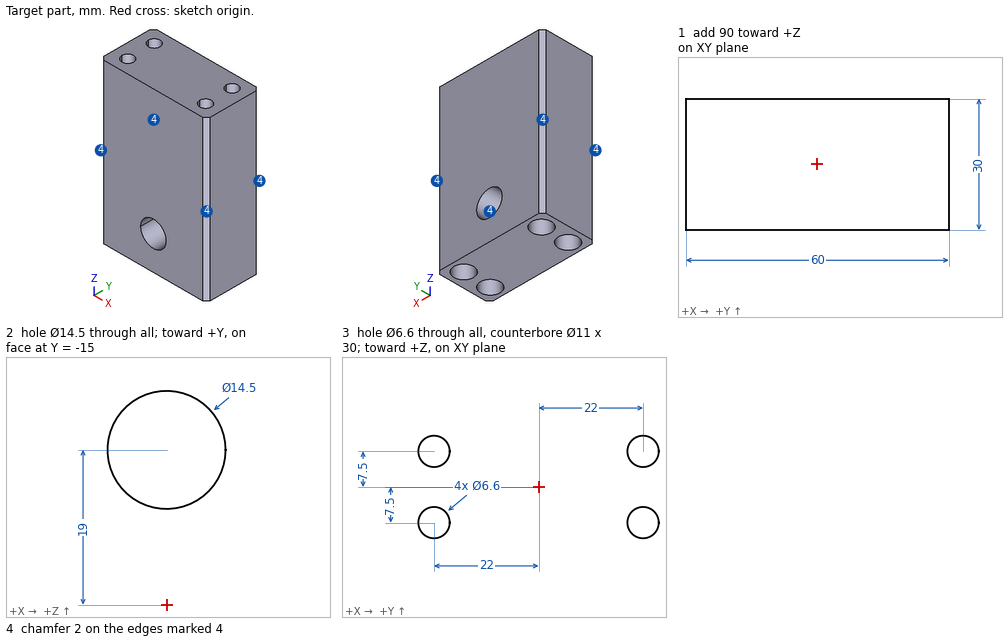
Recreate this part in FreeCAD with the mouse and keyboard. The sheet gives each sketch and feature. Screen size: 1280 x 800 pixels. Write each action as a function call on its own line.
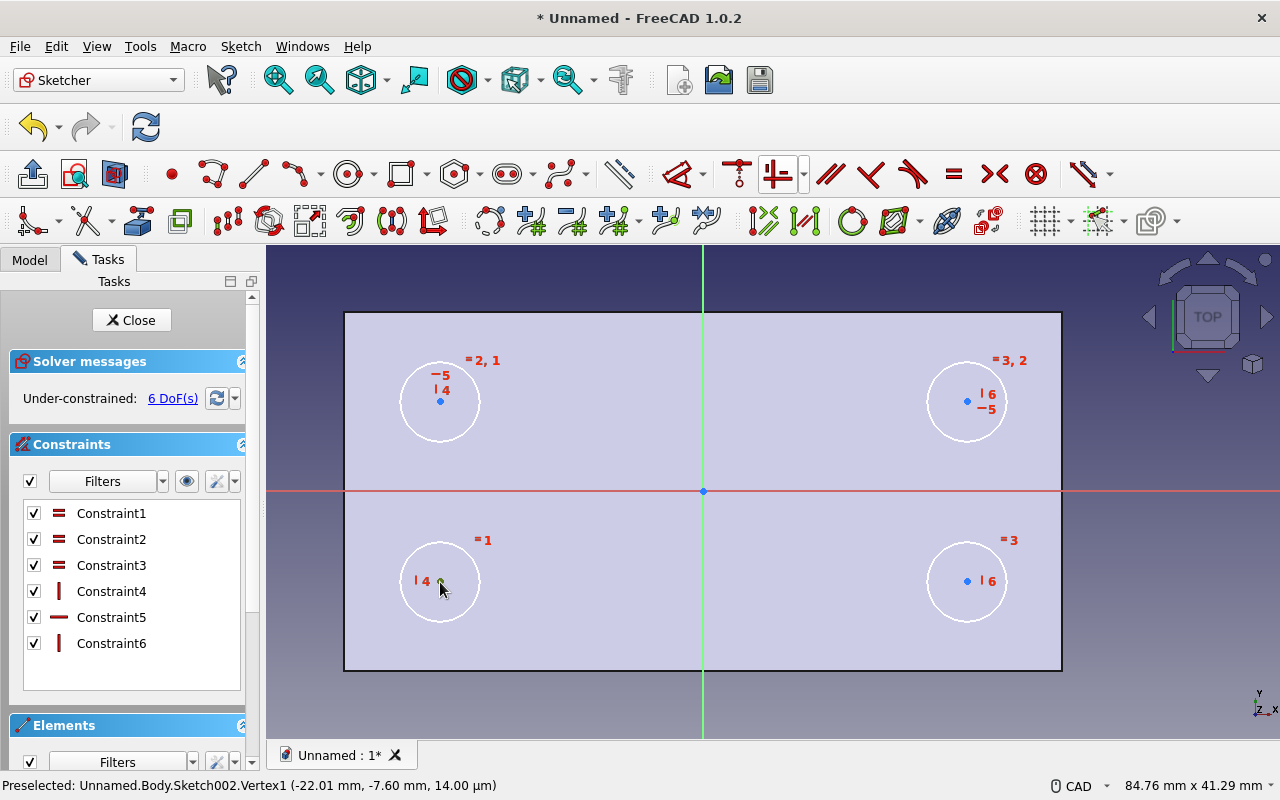
click(967, 582)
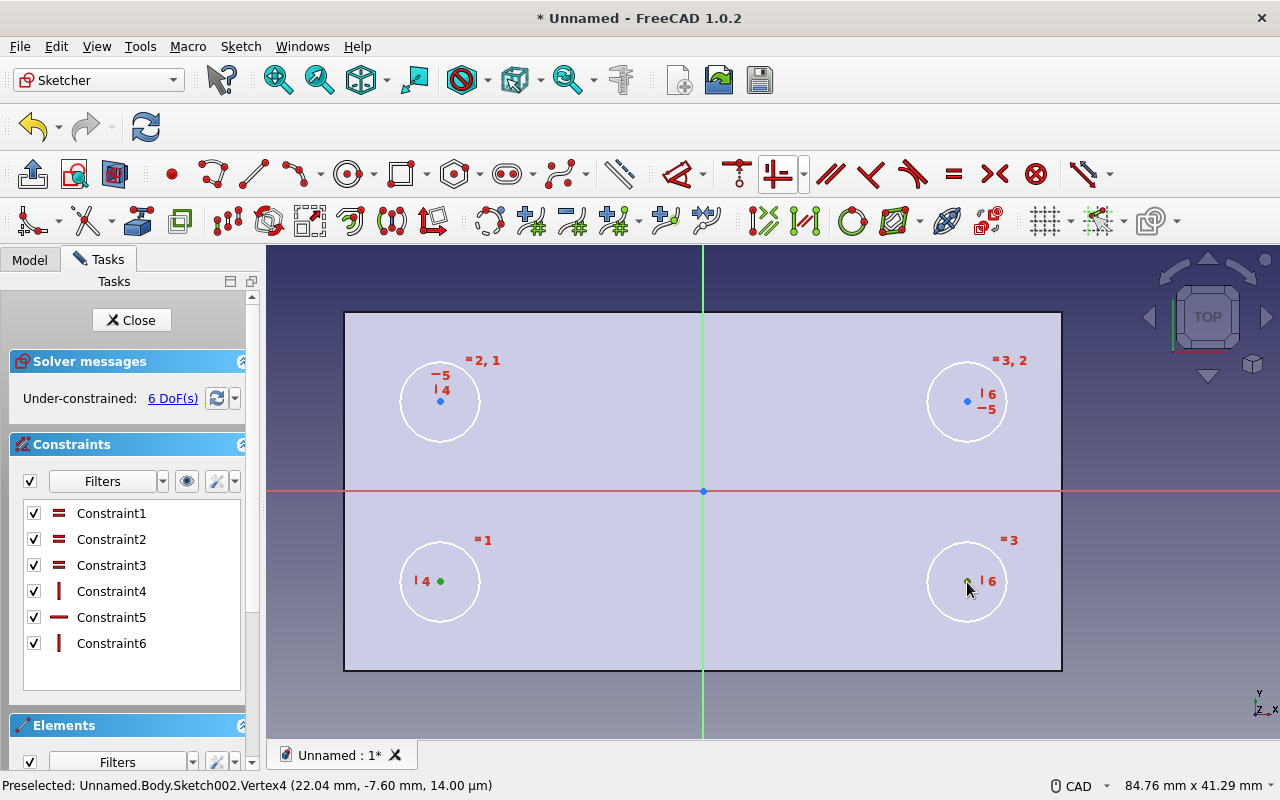
key(h)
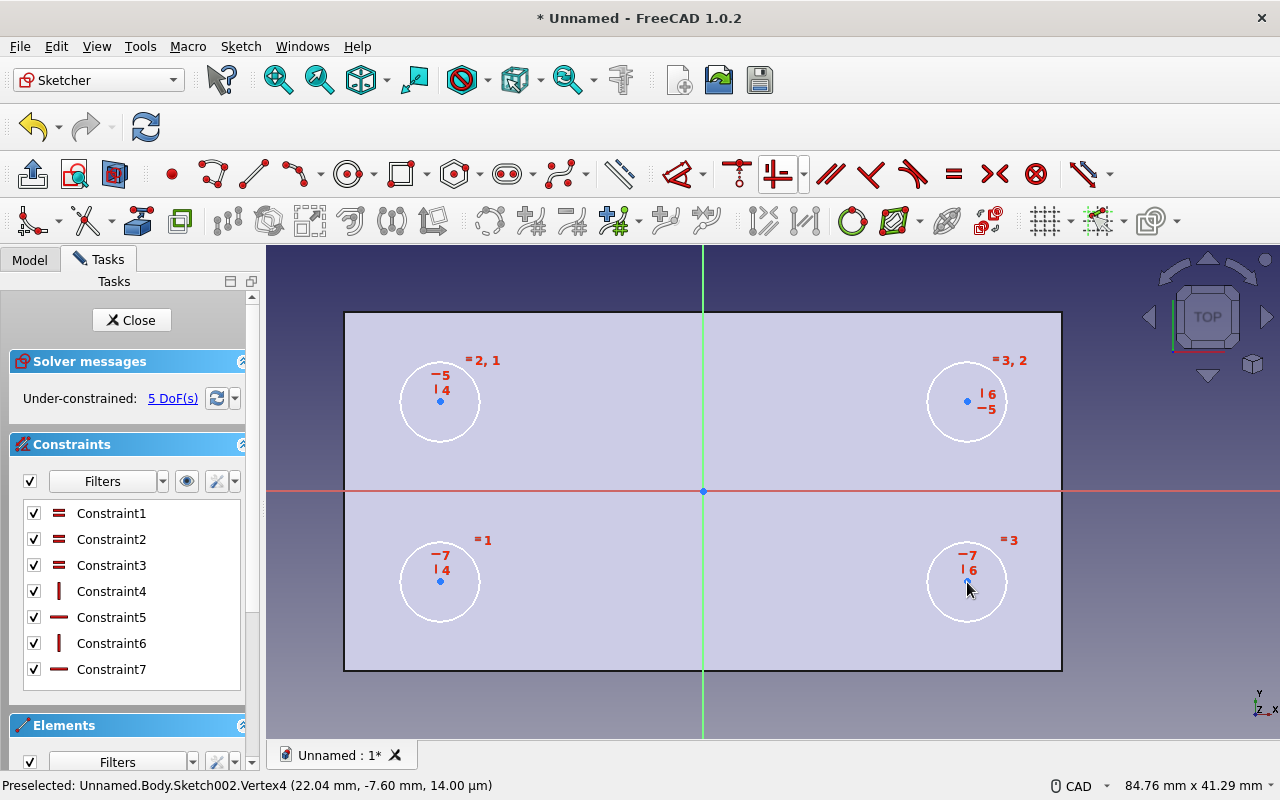
key(d)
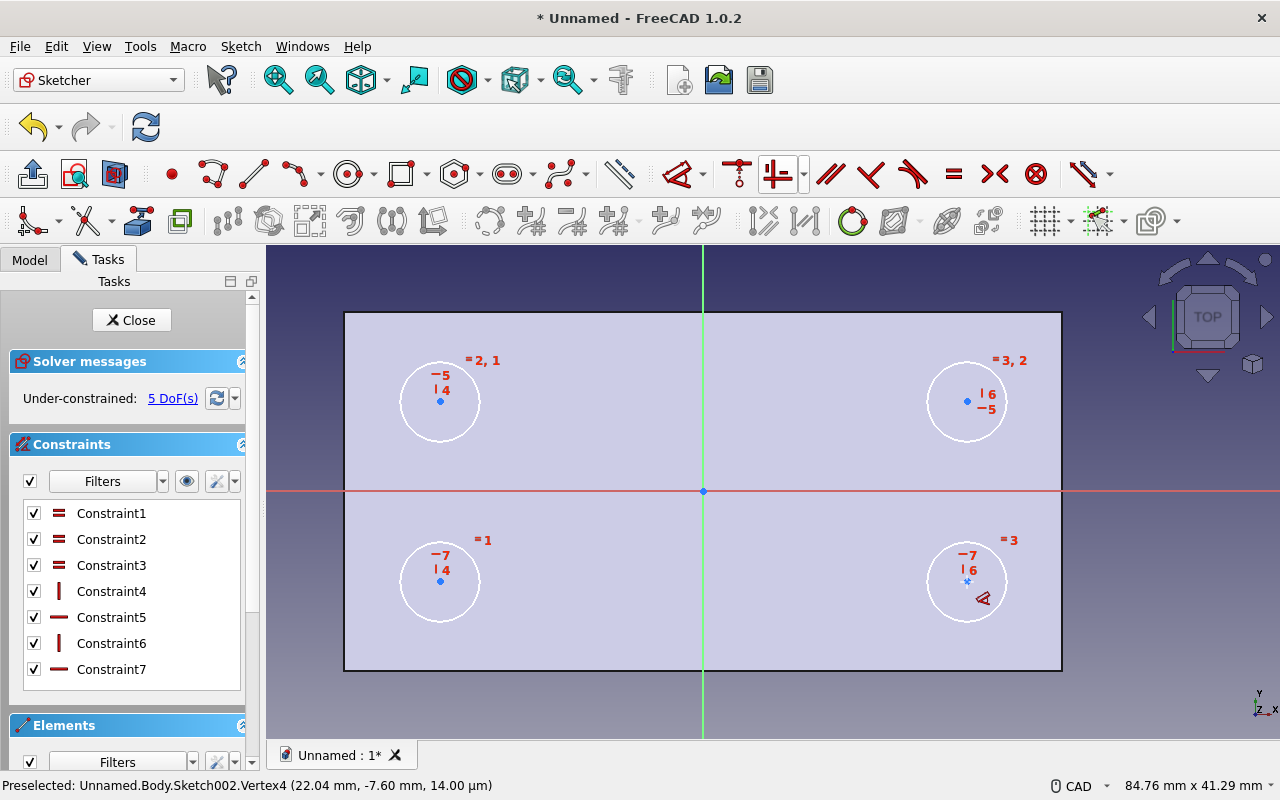
click(468, 554)
click(491, 531)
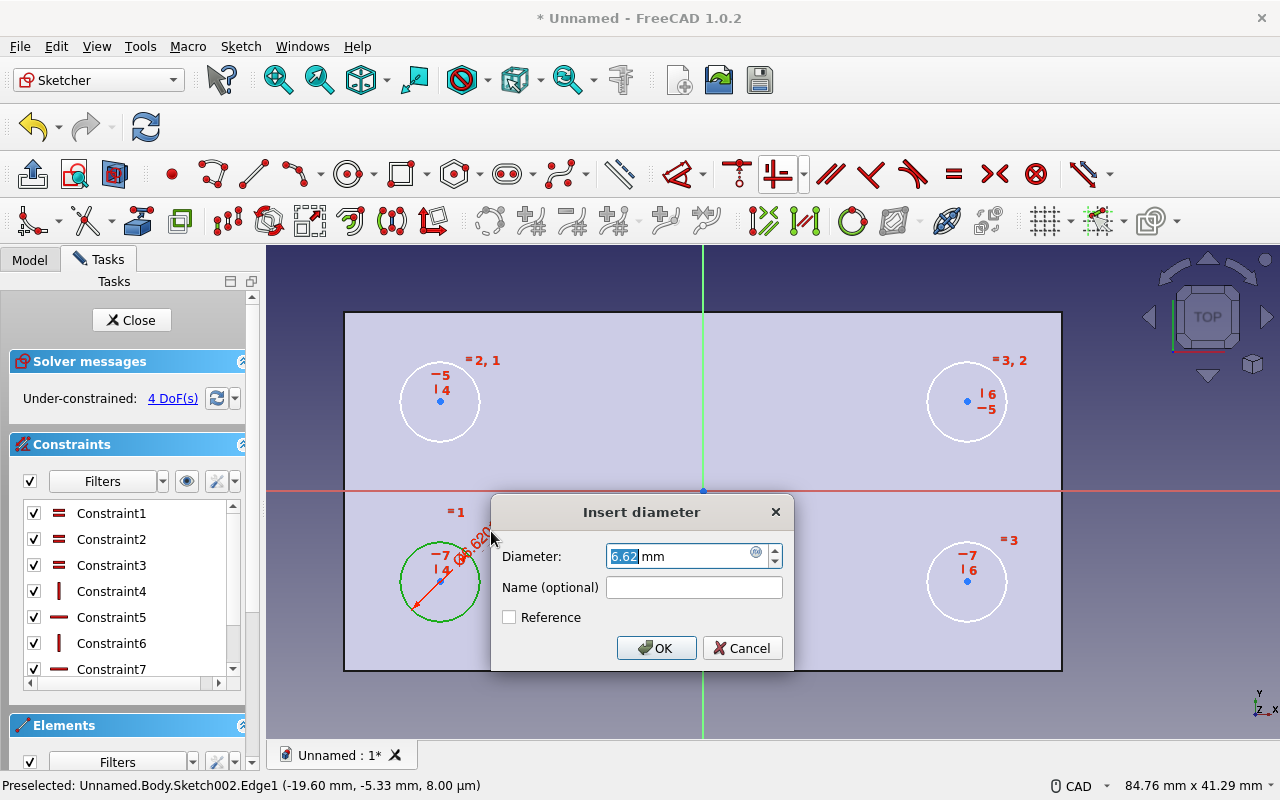
text(6.6)
key(Return)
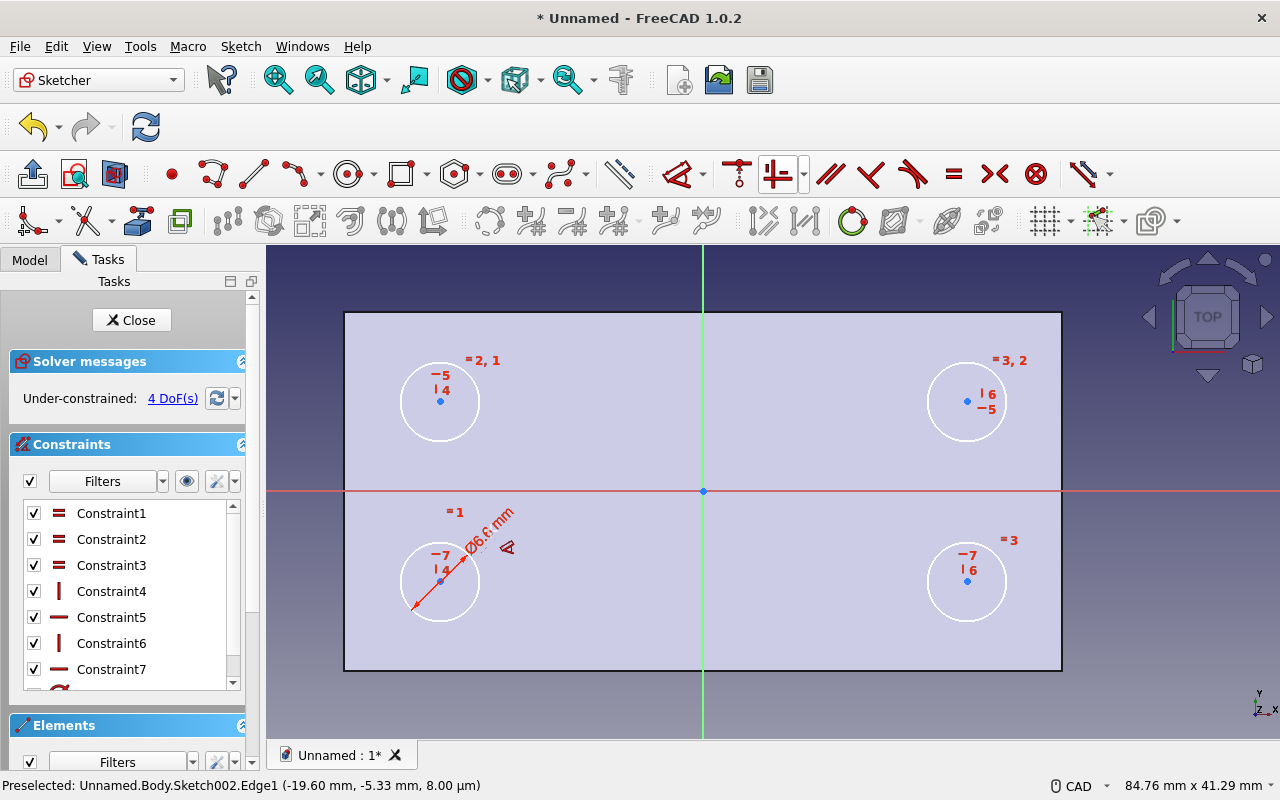
click(440, 582)
click(572, 616)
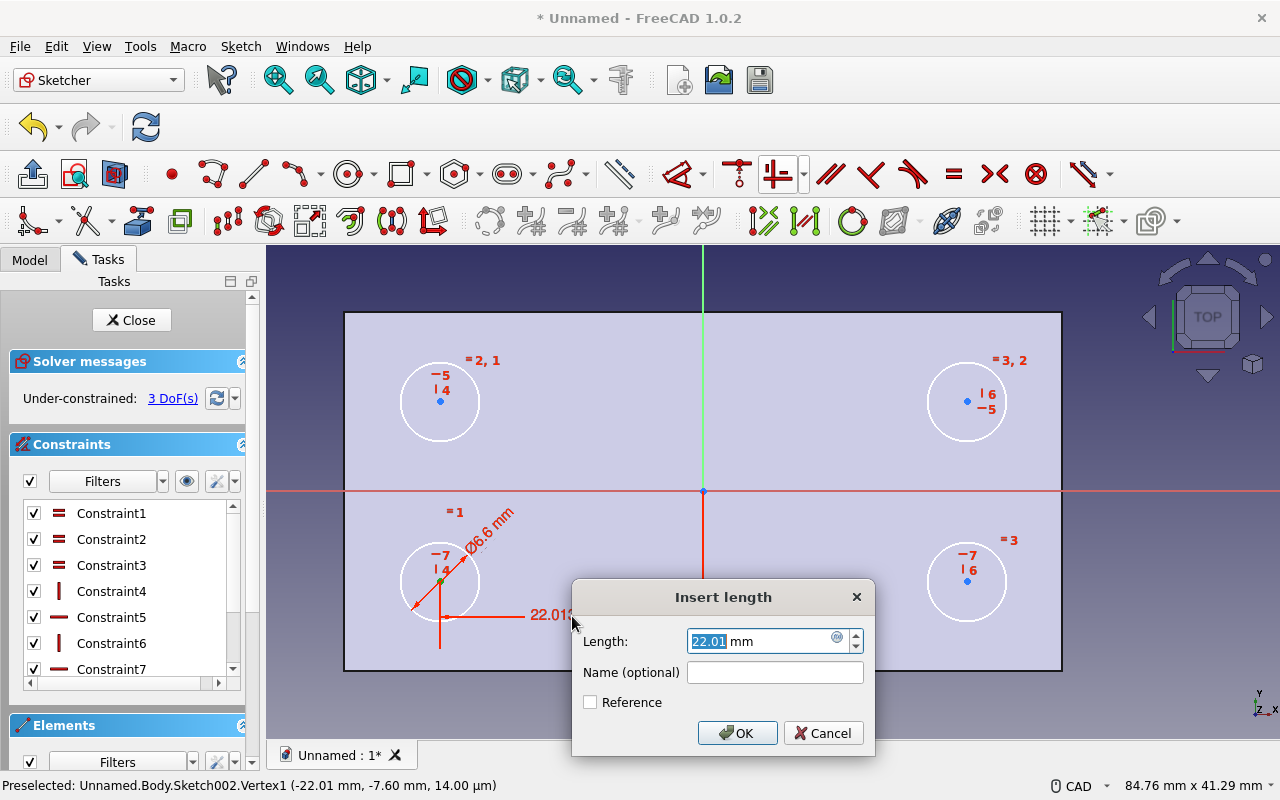
text(22)
key(Return)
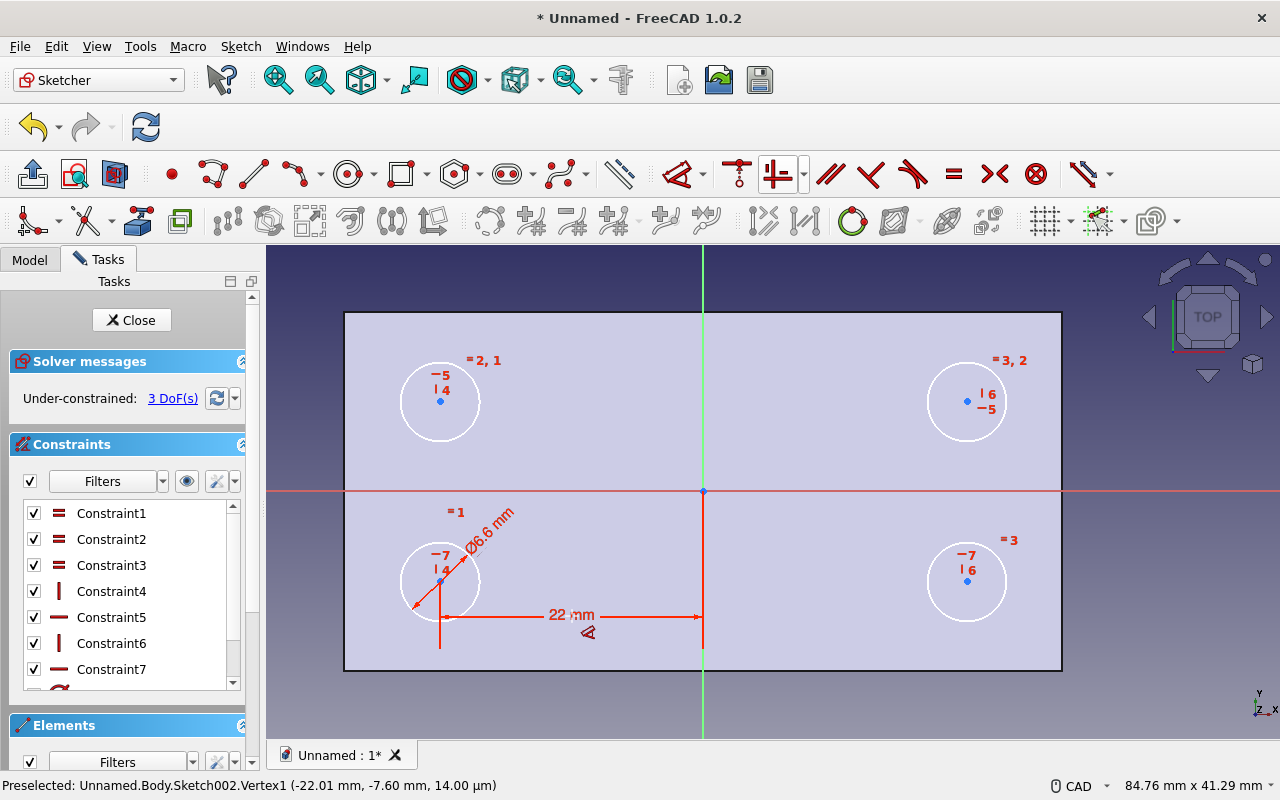
click(967, 402)
click(835, 368)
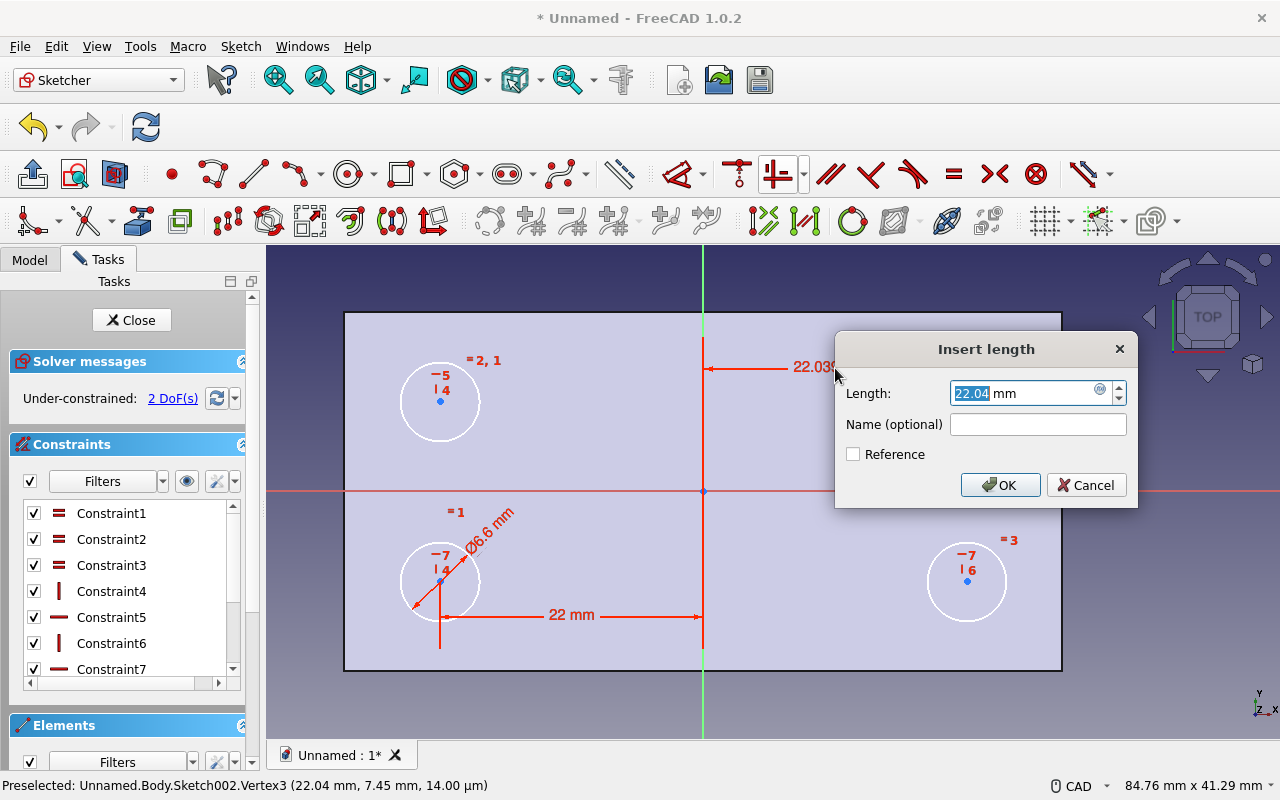
text(22)
key(Return)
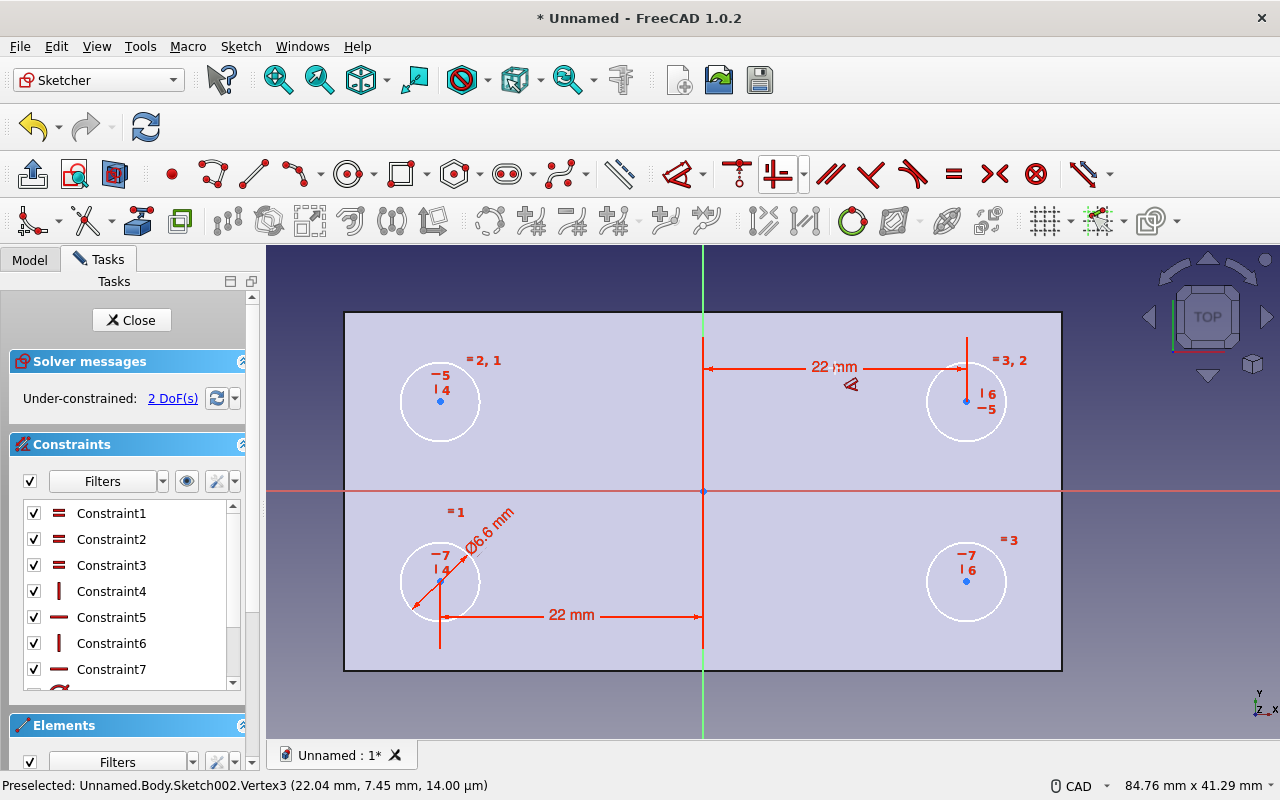
click(440, 582)
click(406, 537)